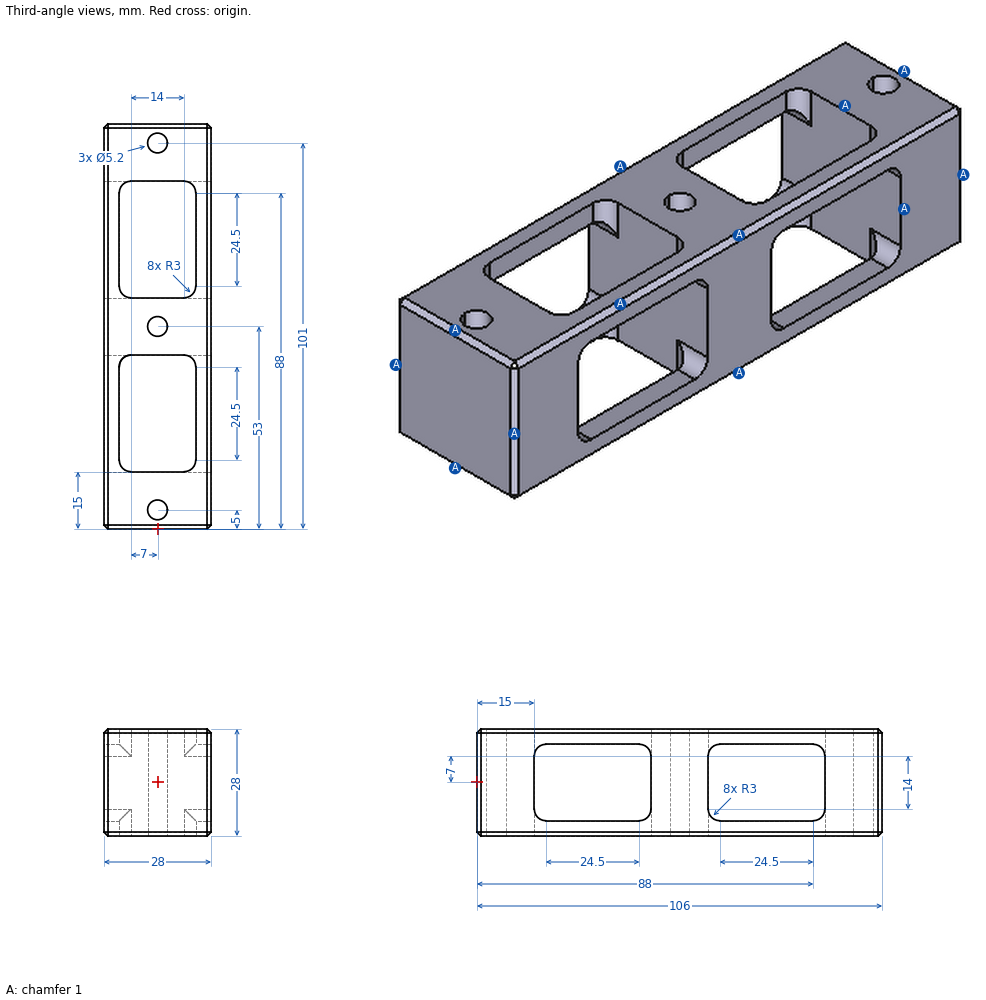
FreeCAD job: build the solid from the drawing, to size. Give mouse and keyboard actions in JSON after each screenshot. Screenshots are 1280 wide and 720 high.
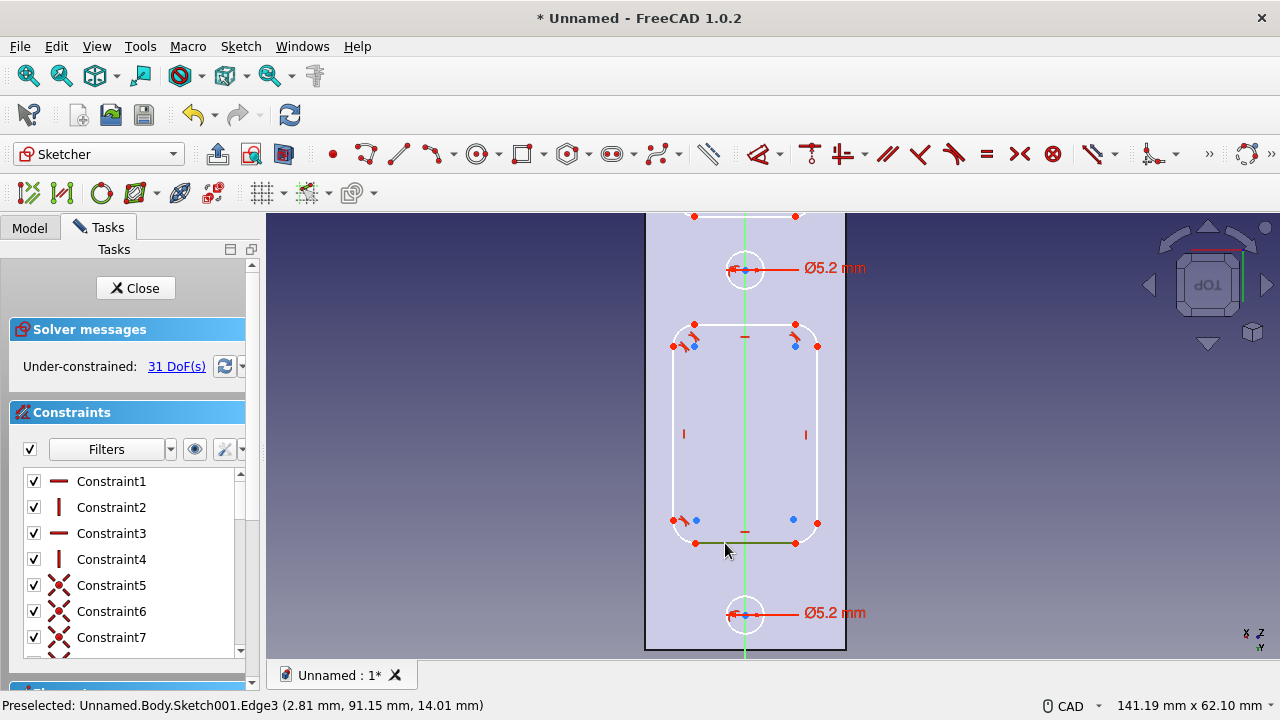
{"action": "scroll", "coordinate": [676, 530], "scroll_direction": "up", "scroll_amount": 2}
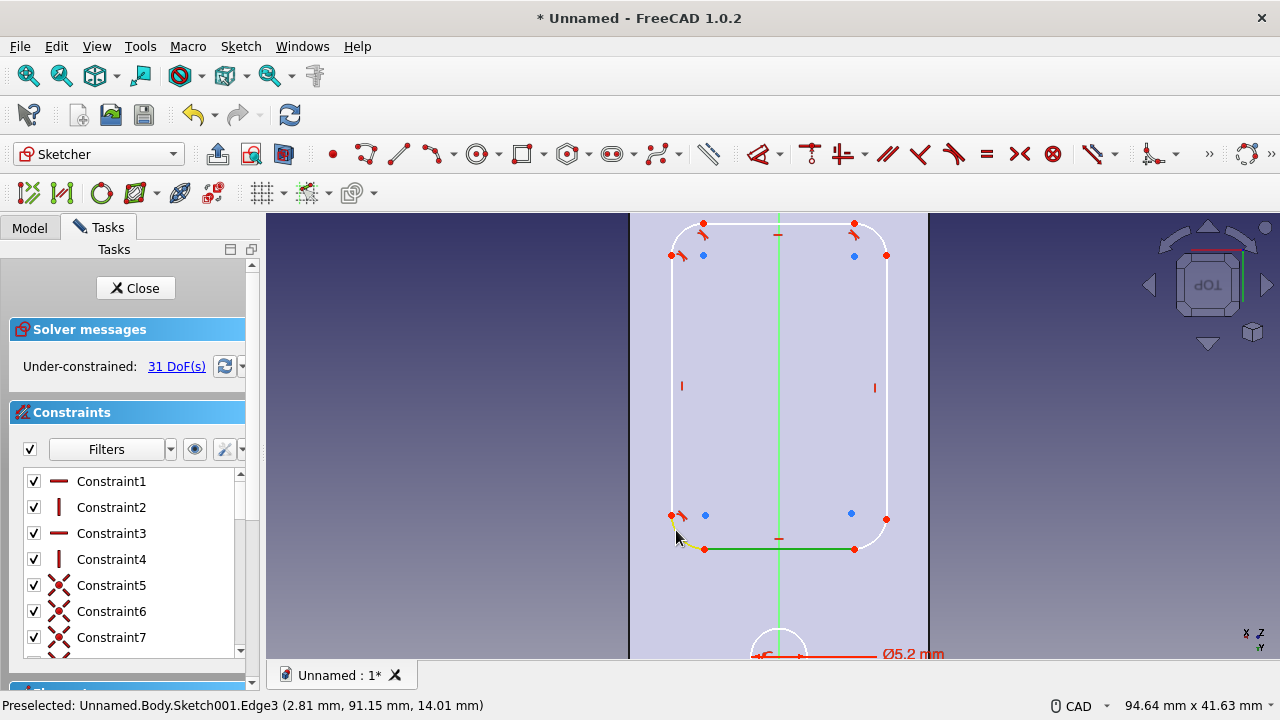
{"action": "left_click", "coordinate": [675, 530]}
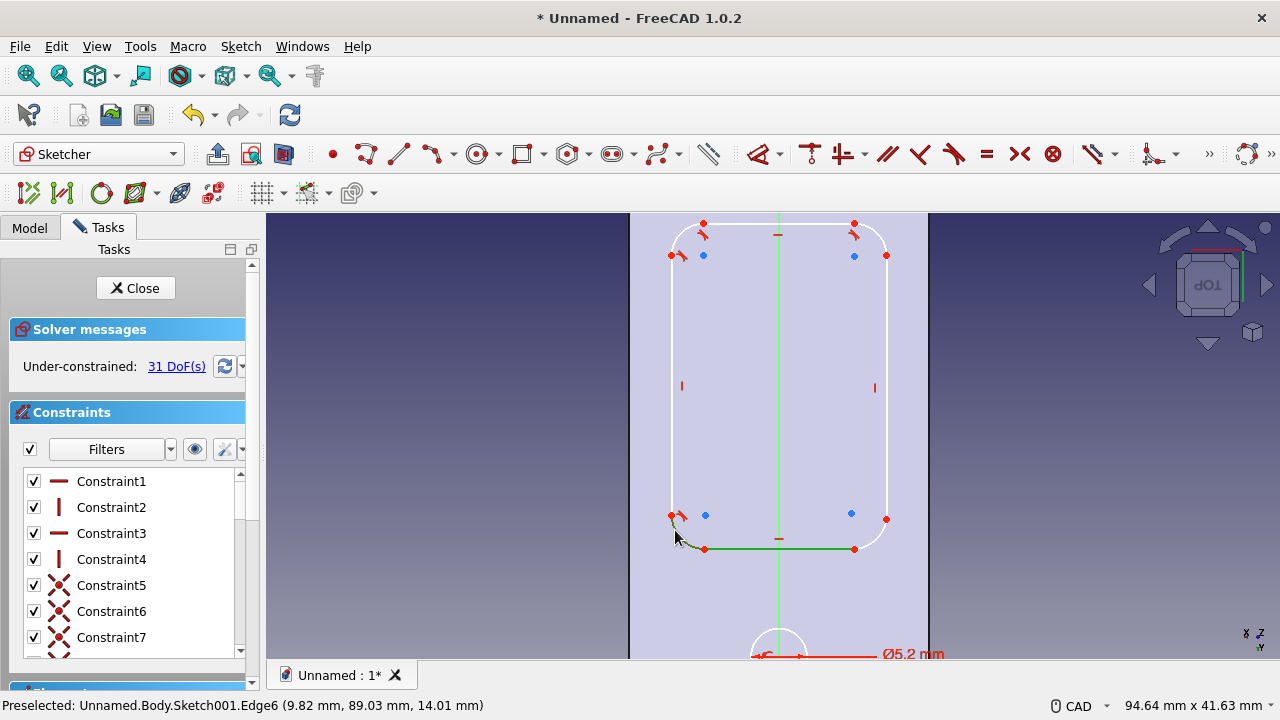
{"action": "left_click", "coordinate": [954, 154]}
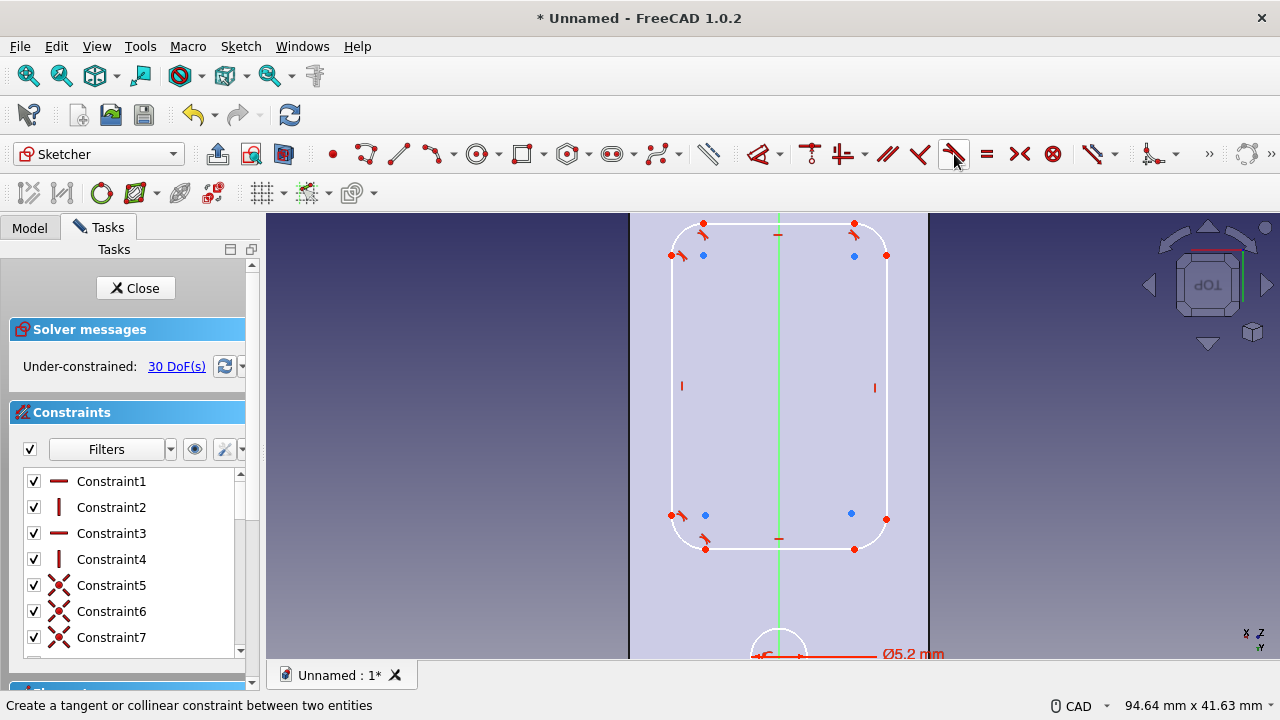
{"action": "left_click", "coordinate": [750, 549]}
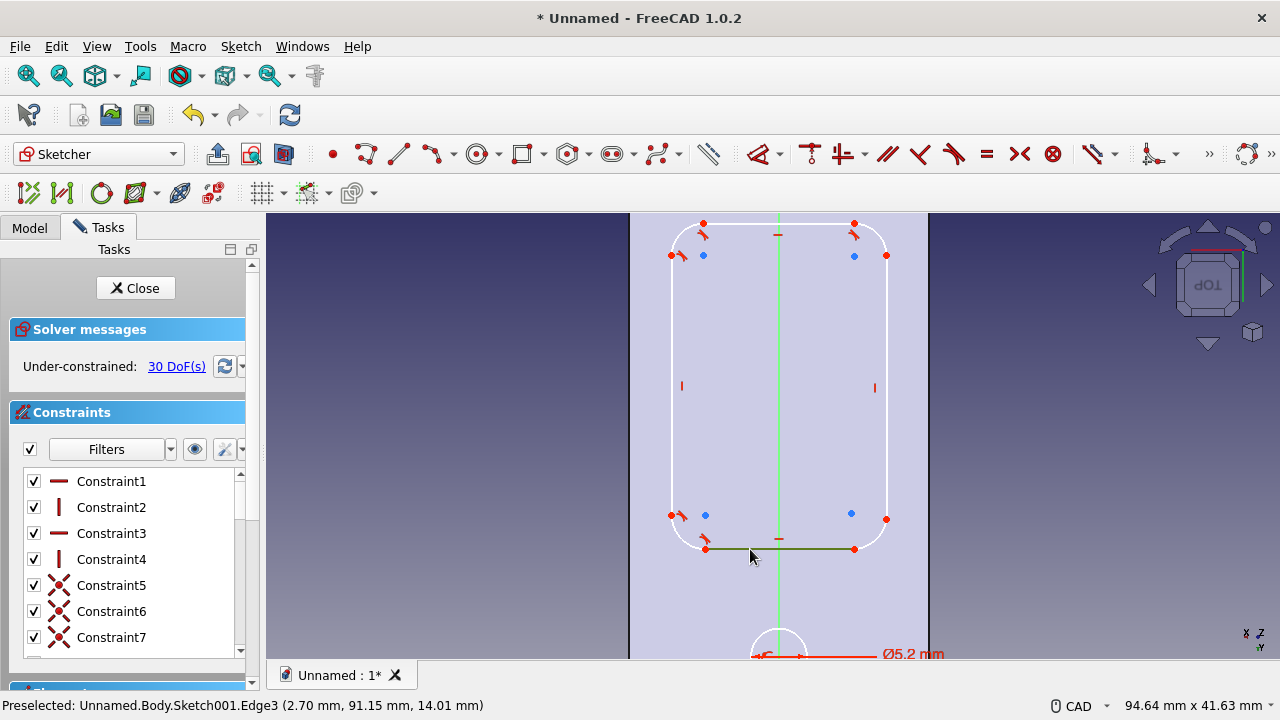
{"action": "left_click", "coordinate": [868, 545]}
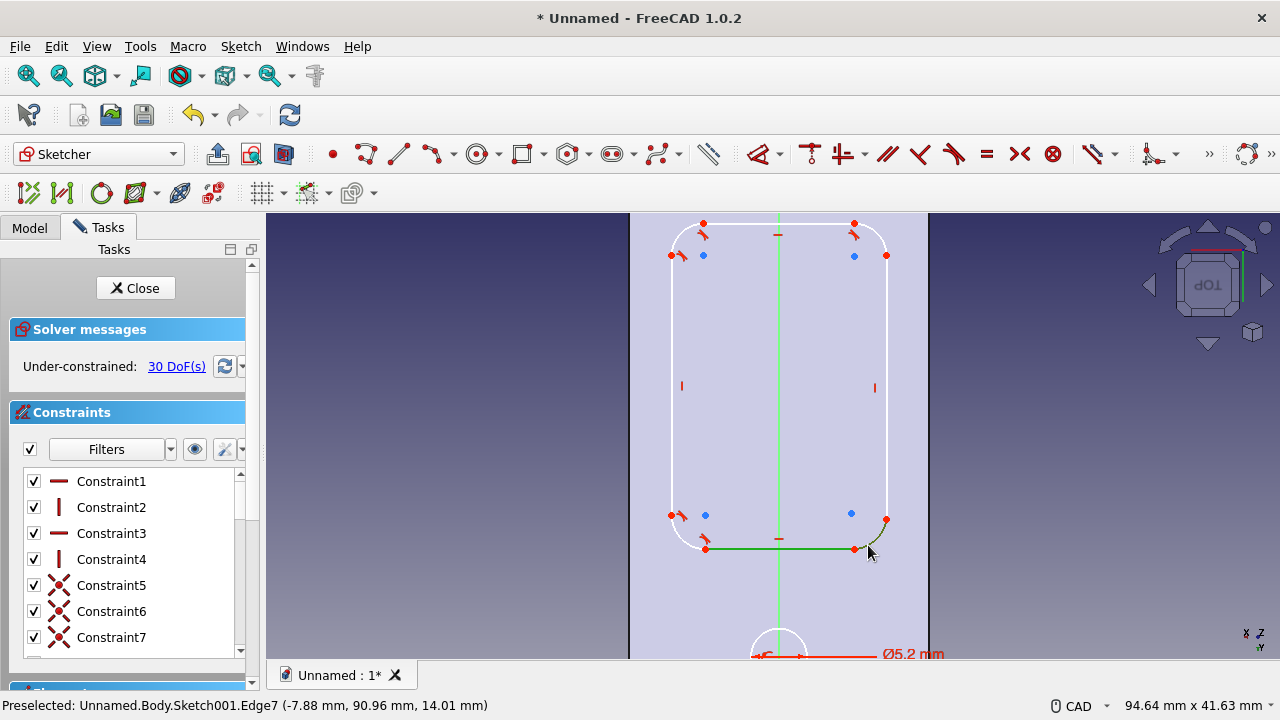
{"action": "left_click", "coordinate": [954, 154]}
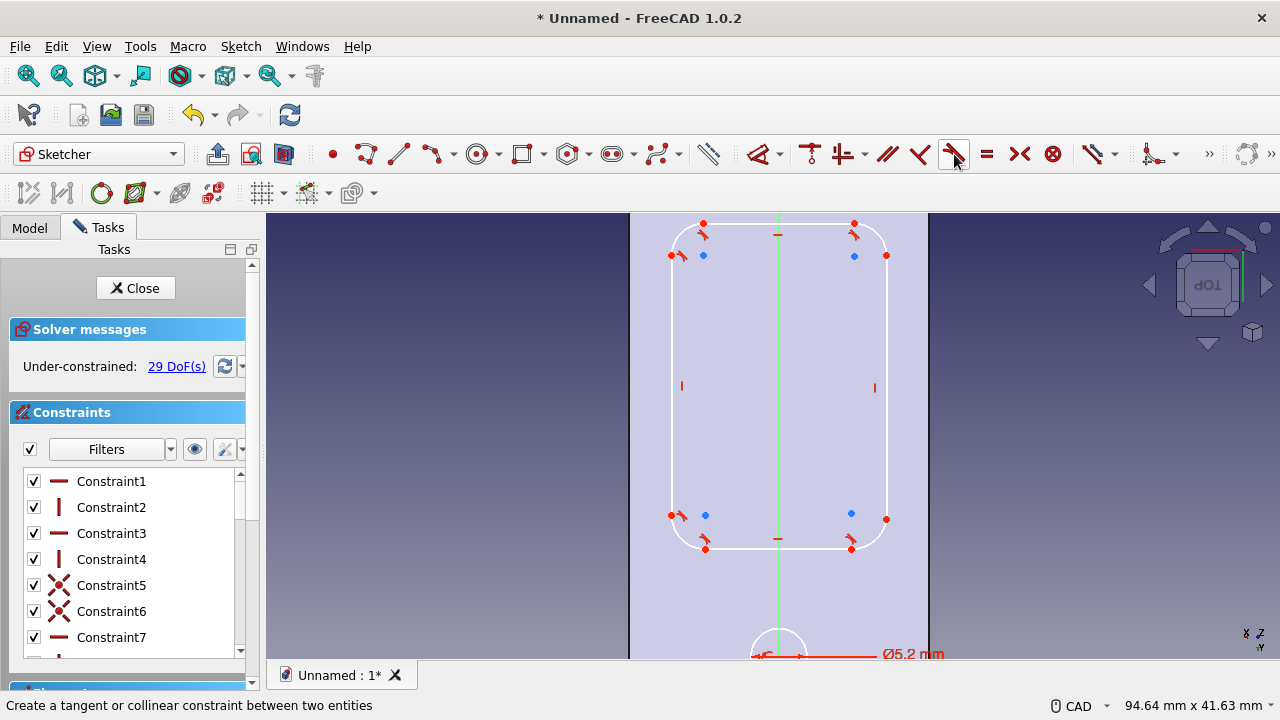
{"action": "scroll", "coordinate": [680, 537], "scroll_direction": "down", "scroll_amount": 7}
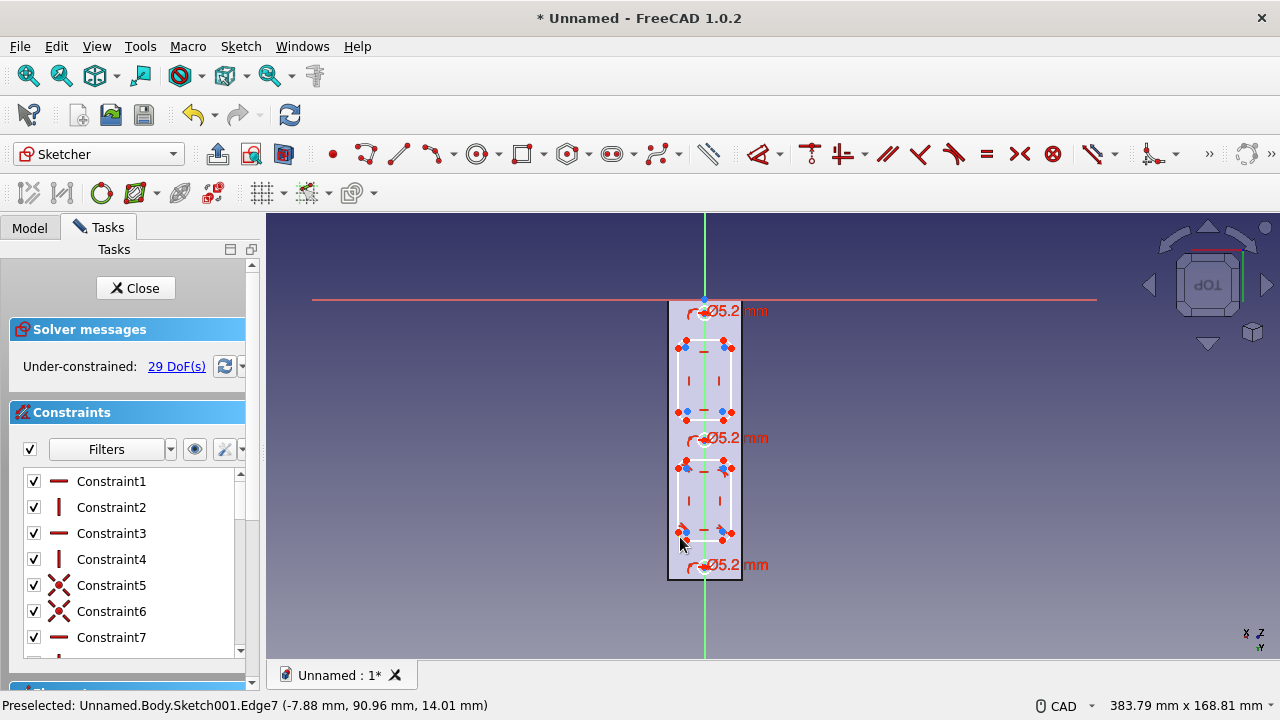
{"action": "left_click", "coordinate": [731, 514]}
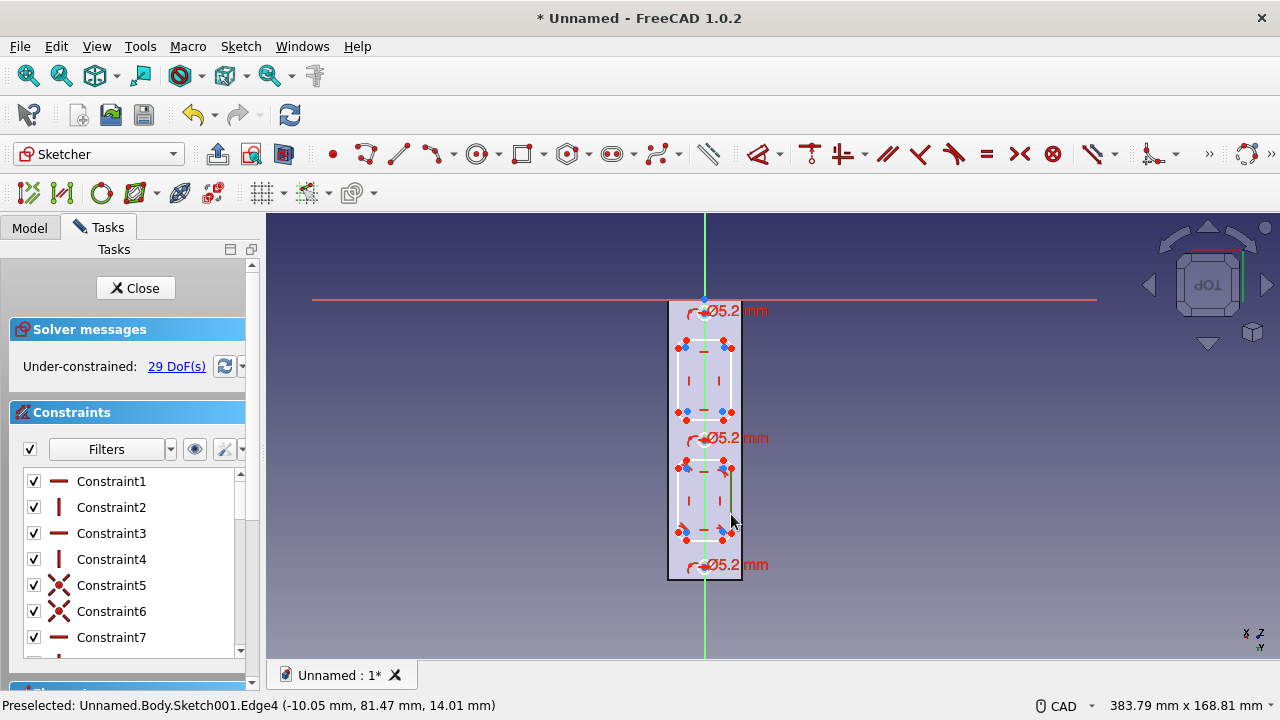
{"action": "scroll", "coordinate": [728, 538], "scroll_direction": "up", "scroll_amount": 5}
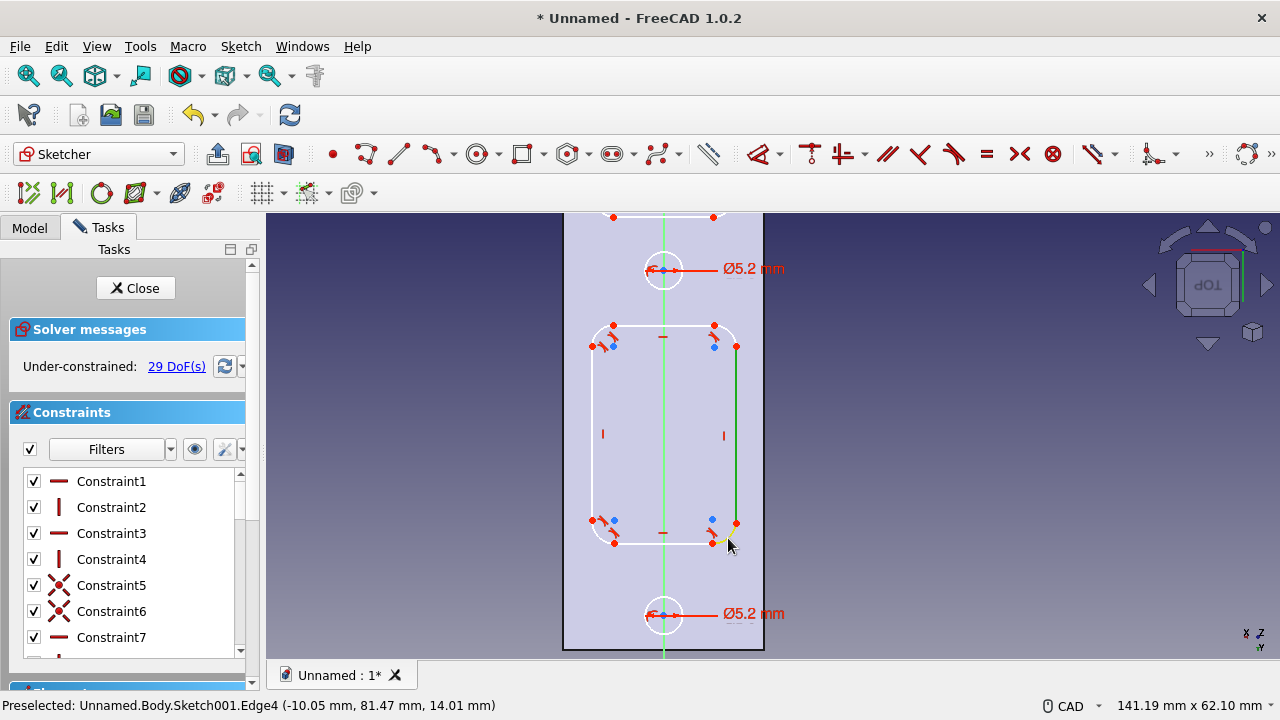
{"action": "left_click", "coordinate": [728, 538]}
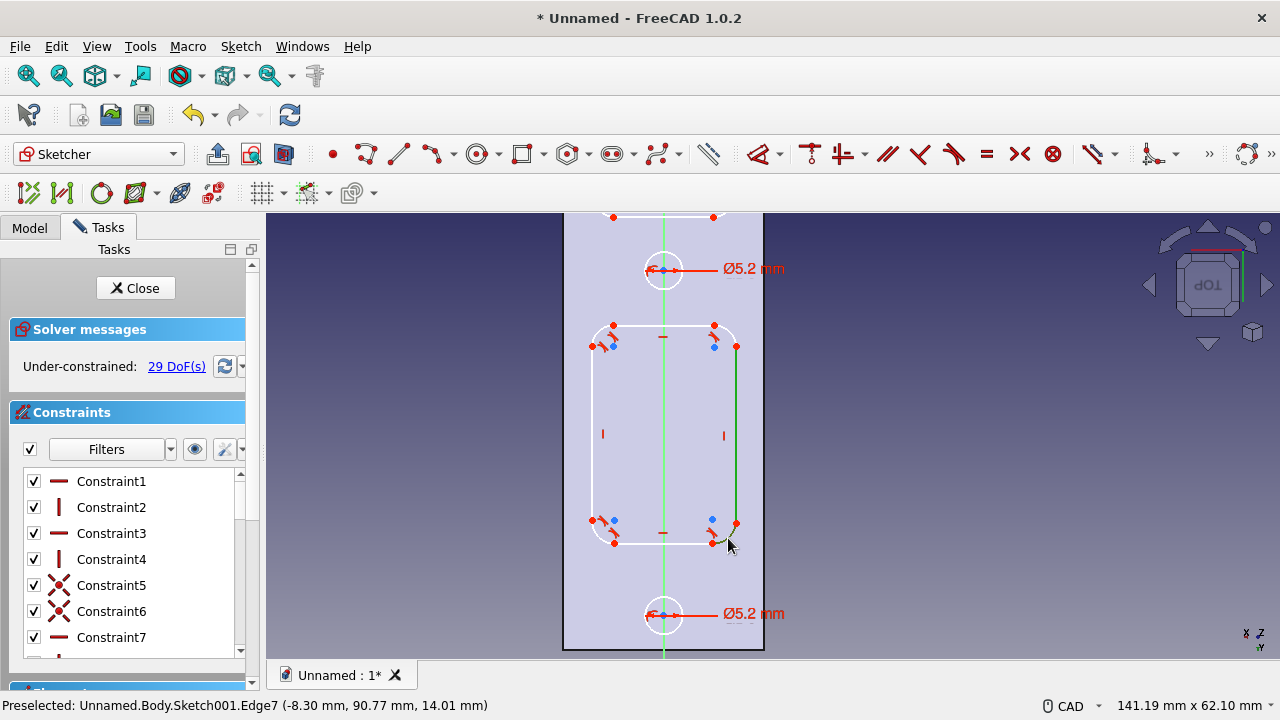
{"action": "left_click", "coordinate": [954, 154]}